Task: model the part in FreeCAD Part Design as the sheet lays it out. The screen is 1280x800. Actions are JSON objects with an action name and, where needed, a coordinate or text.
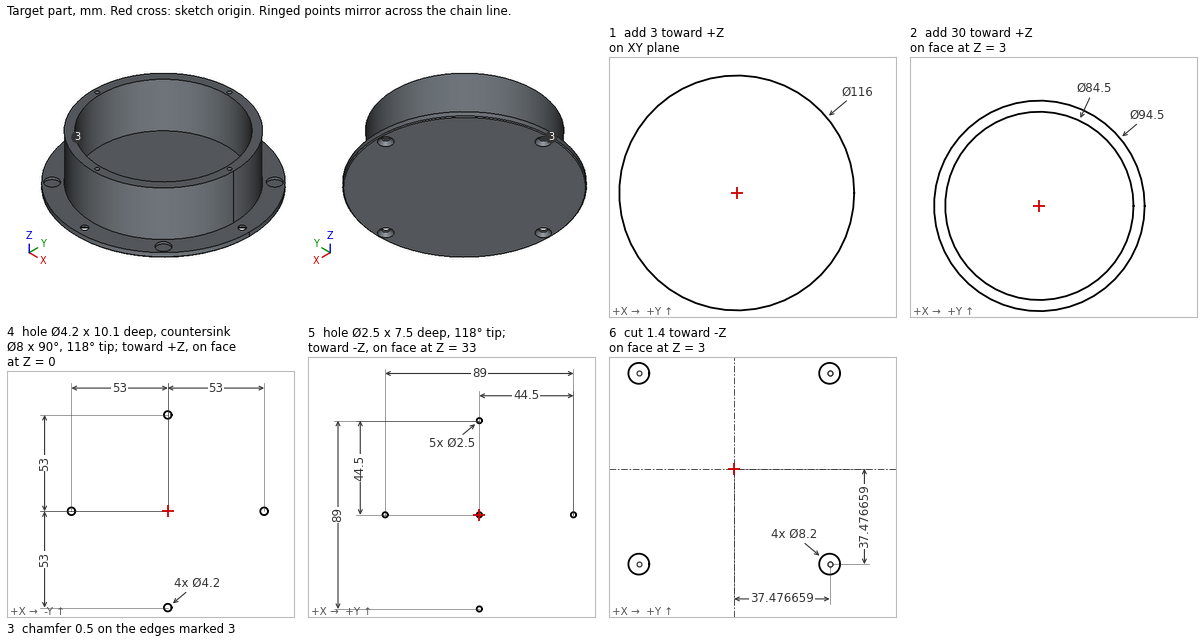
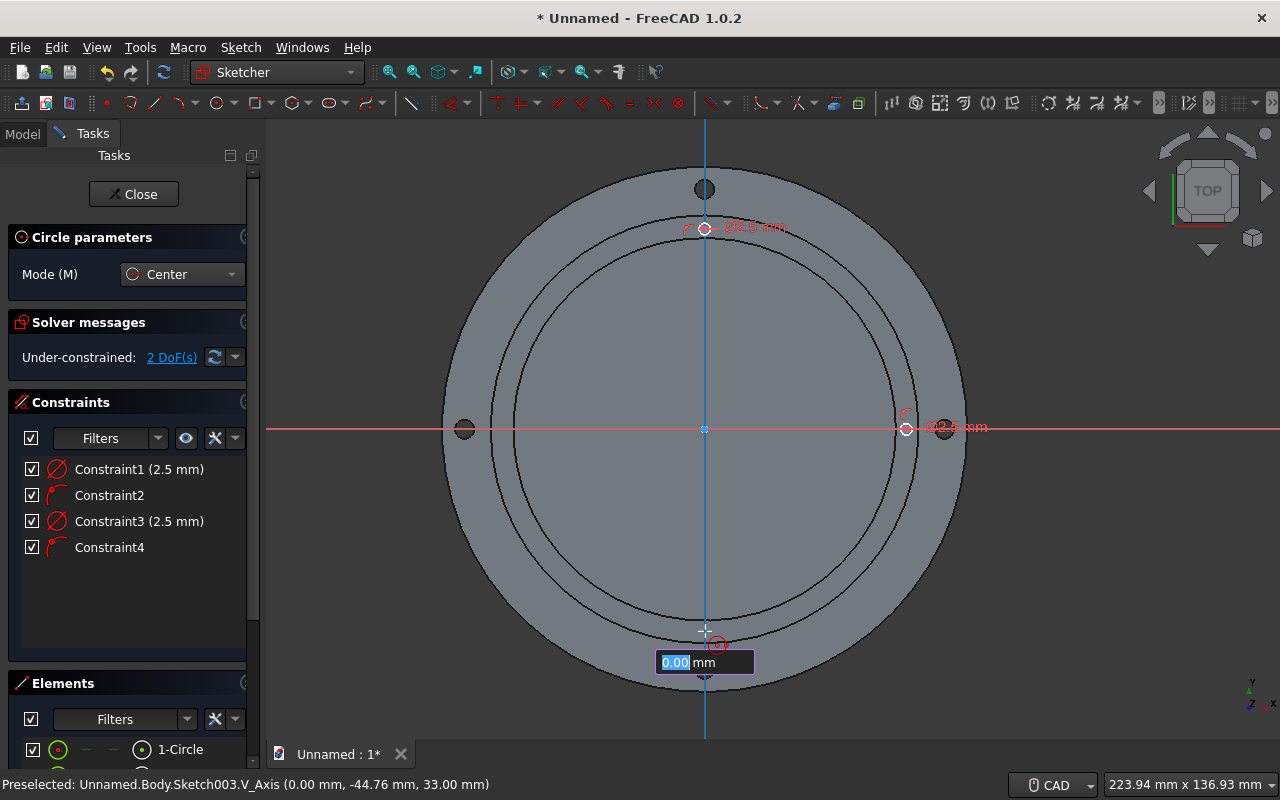
{"action": "scroll", "coordinate": [710, 629], "scroll_direction": "up", "scroll_amount": 6}
{"action": "mouse_move", "coordinate": [709, 627]}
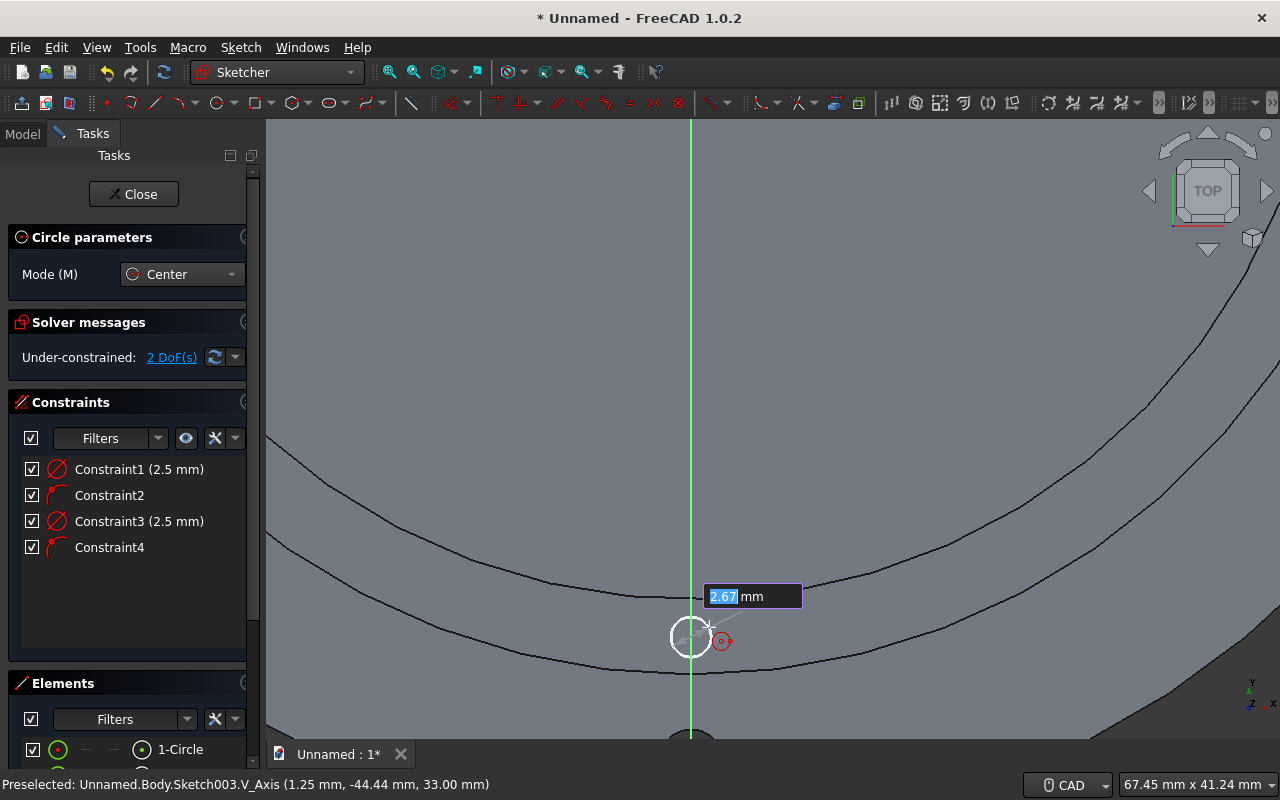
{"action": "type", "text": "2.5"}
{"action": "key", "text": "Return"}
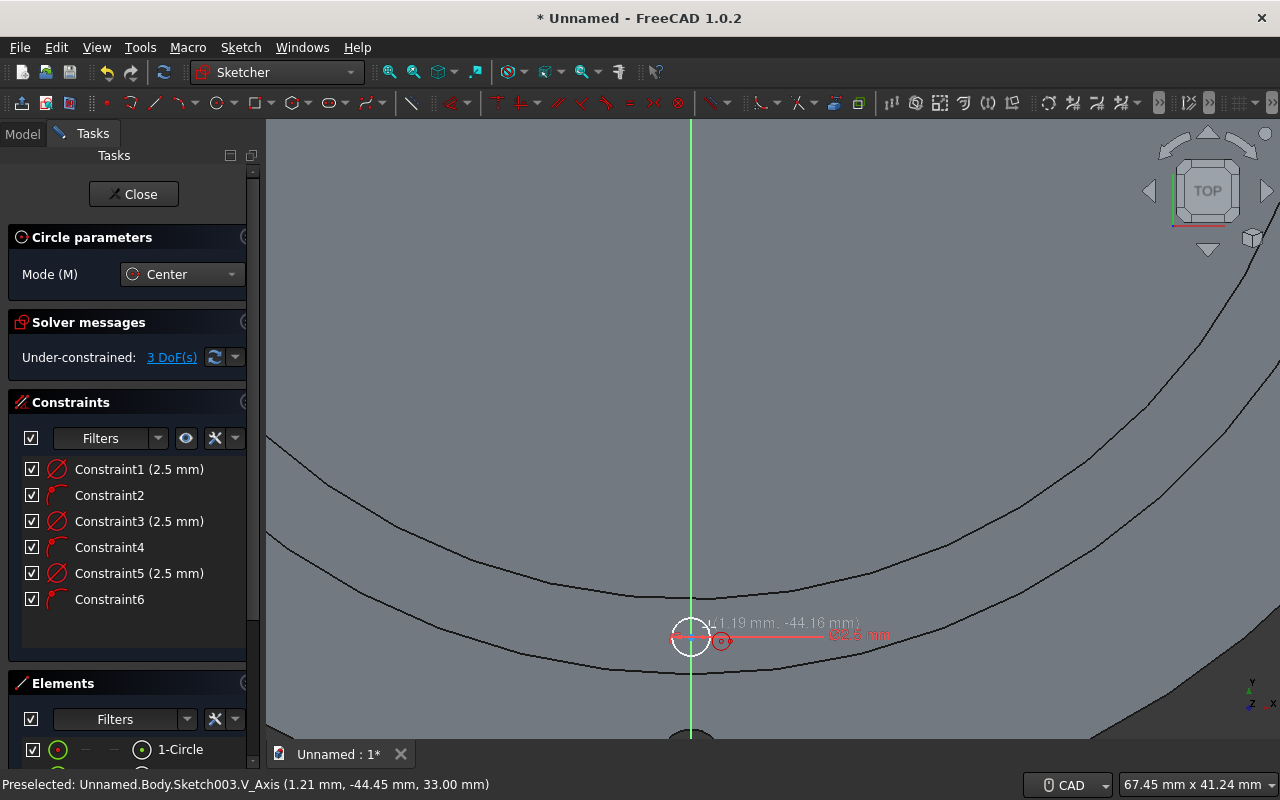
{"action": "scroll", "coordinate": [710, 629], "scroll_direction": "down", "scroll_amount": 6}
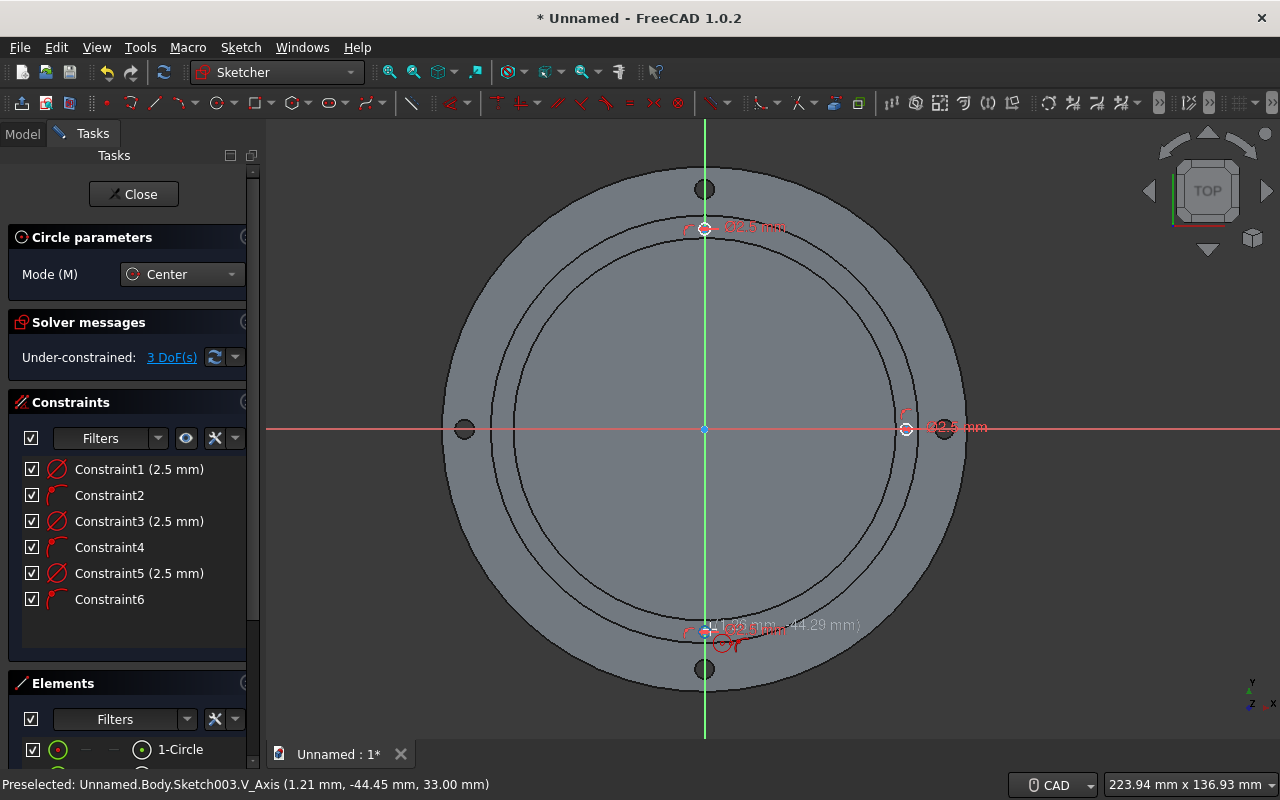
{"action": "scroll", "coordinate": [503, 429], "scroll_direction": "up", "scroll_amount": 7}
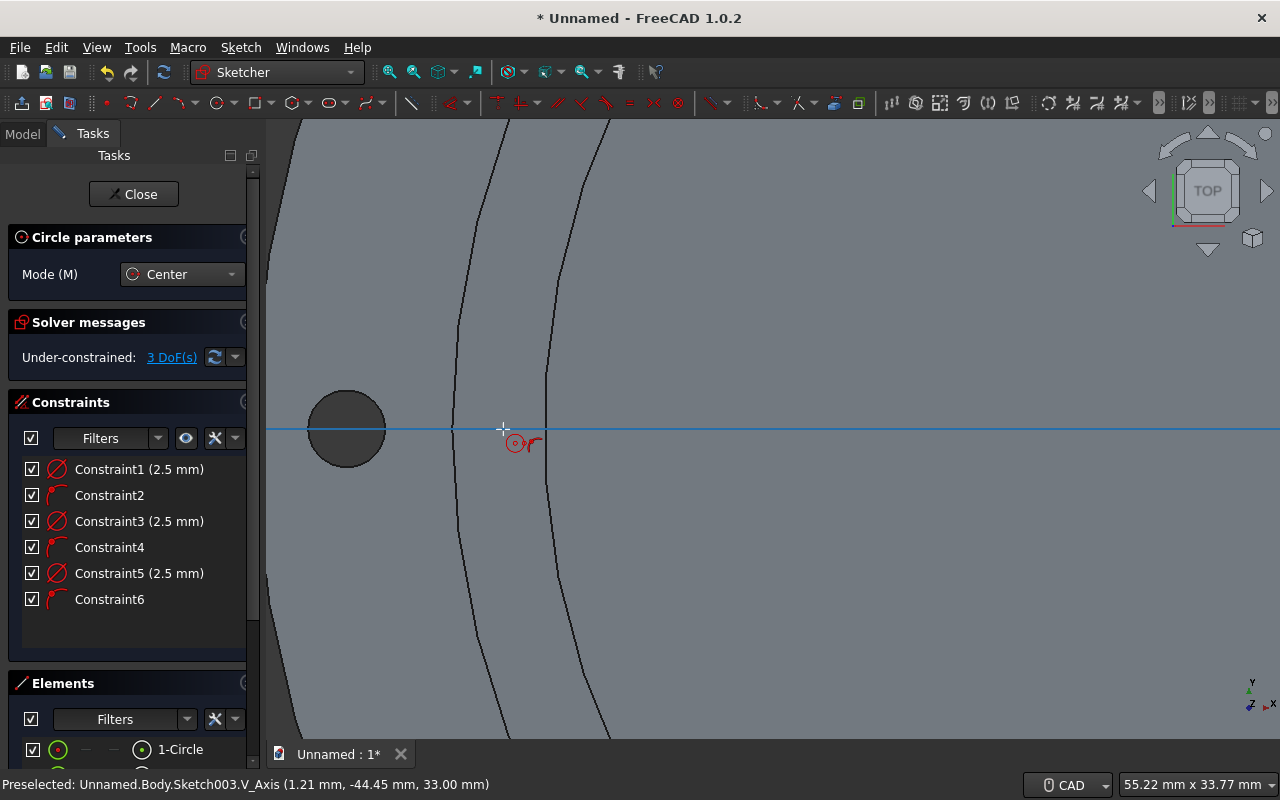
{"action": "scroll", "coordinate": [503, 429], "scroll_direction": "down", "scroll_amount": 7}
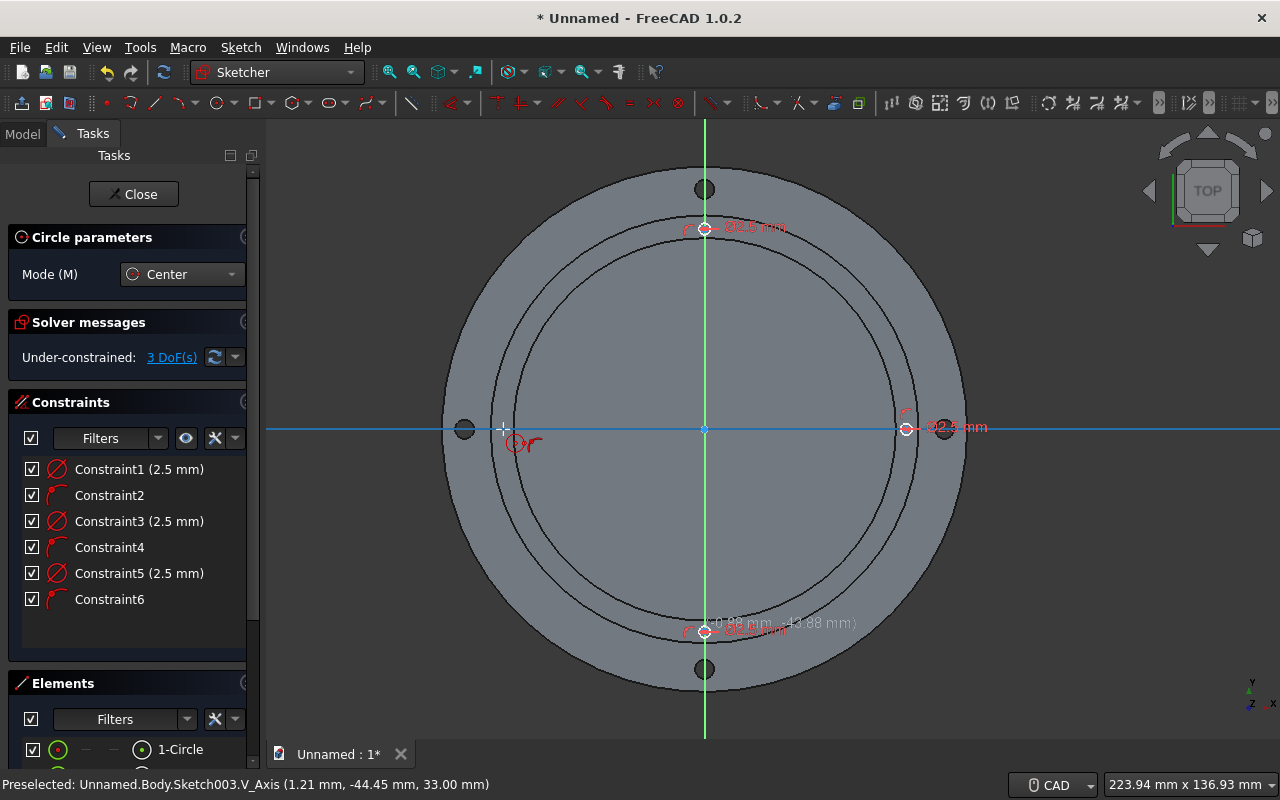
{"action": "left_click", "coordinate": [503, 429]}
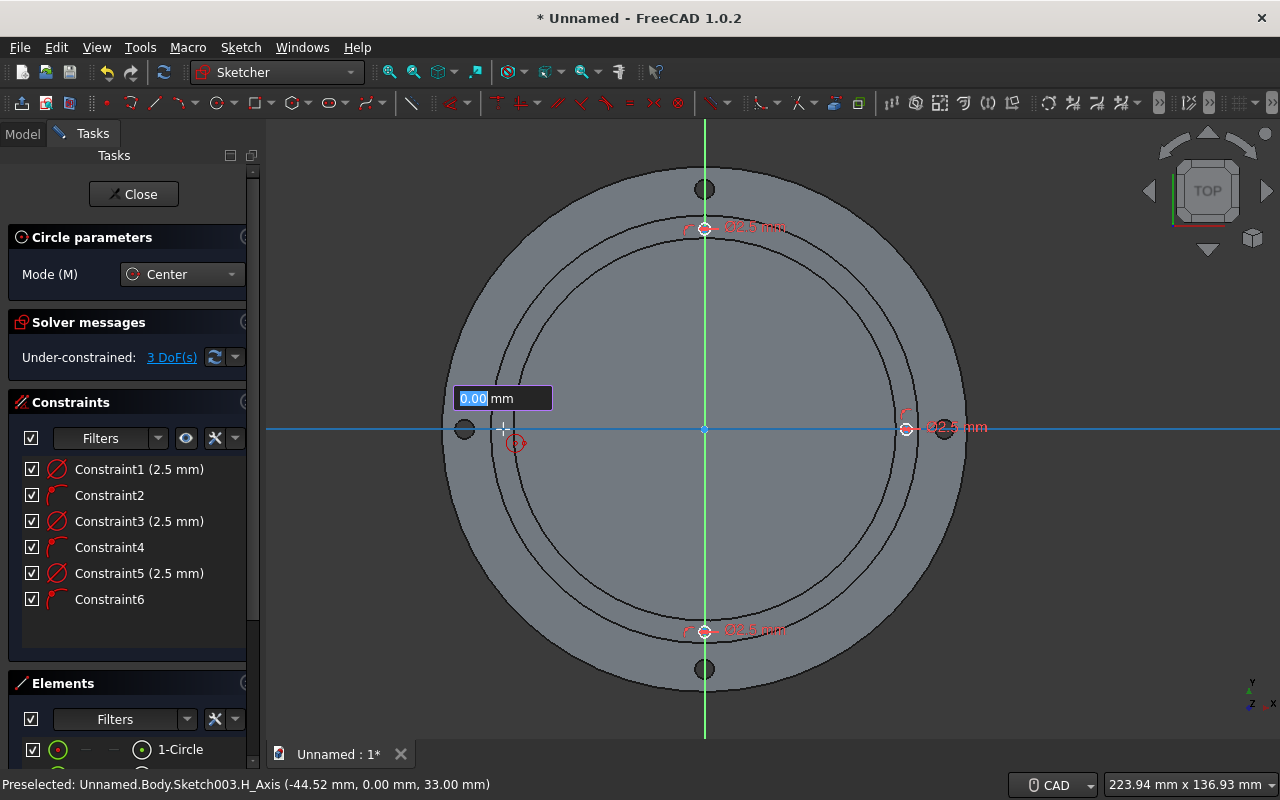
{"action": "scroll", "coordinate": [501, 435], "scroll_direction": "up", "scroll_amount": 6}
{"action": "mouse_move", "coordinate": [501, 433]}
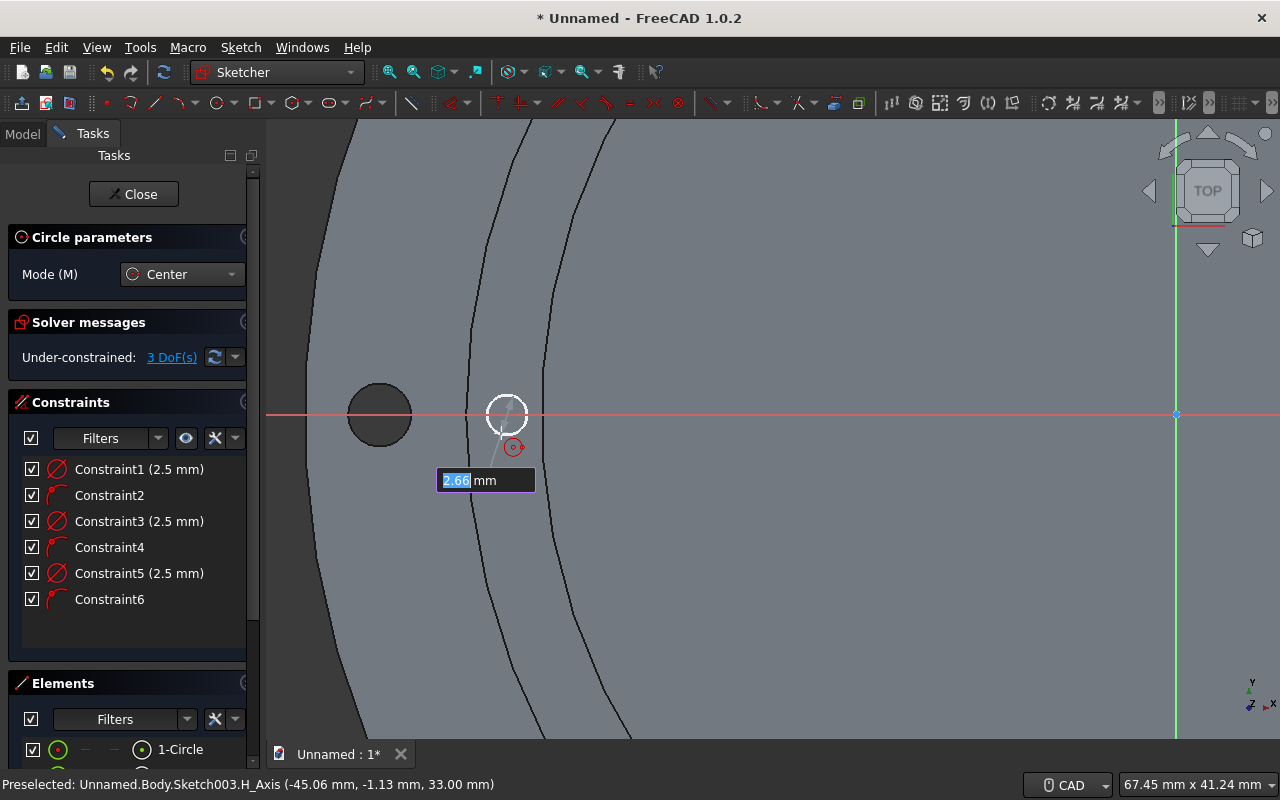
{"action": "type", "text": "2.5"}
{"action": "key", "text": "Return"}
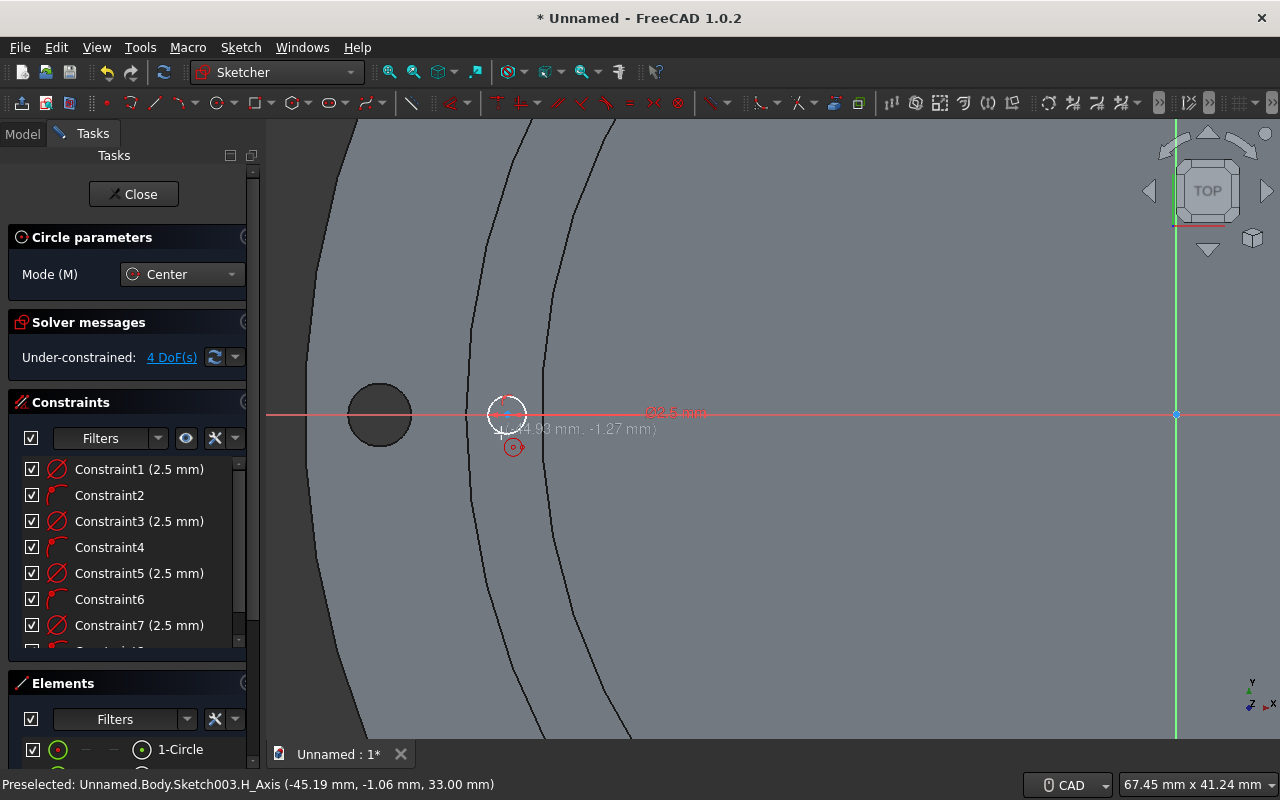
{"action": "scroll", "coordinate": [501, 435], "scroll_direction": "down", "scroll_amount": 6}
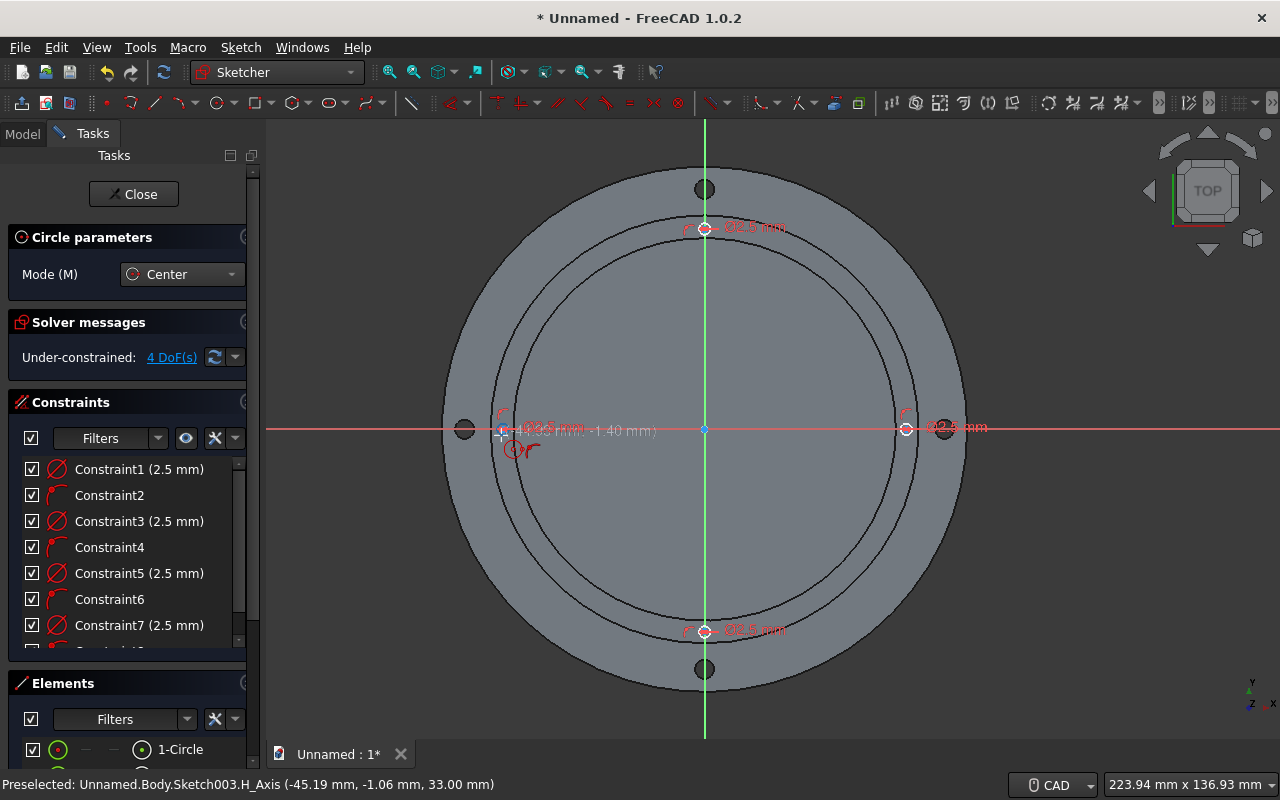
{"action": "scroll", "coordinate": [705, 429], "scroll_direction": "up", "scroll_amount": 7}